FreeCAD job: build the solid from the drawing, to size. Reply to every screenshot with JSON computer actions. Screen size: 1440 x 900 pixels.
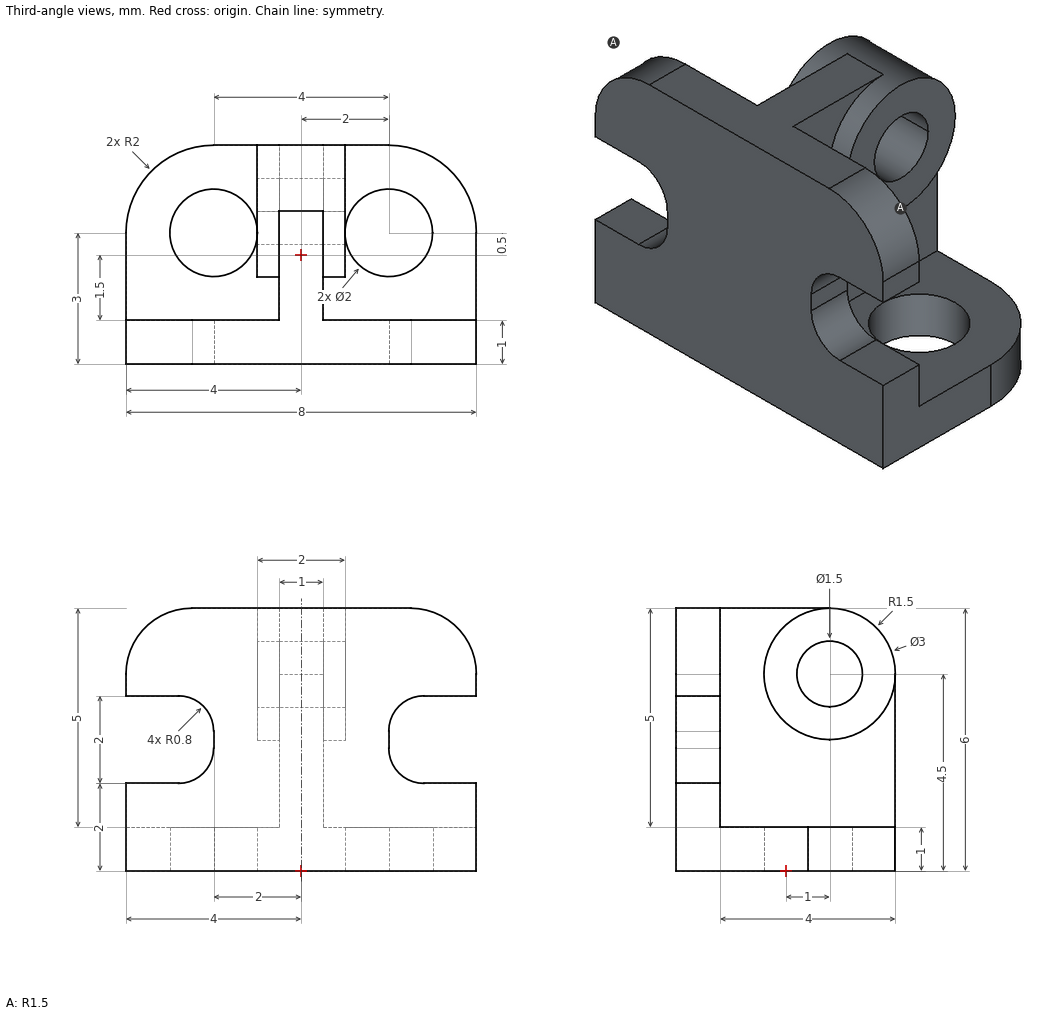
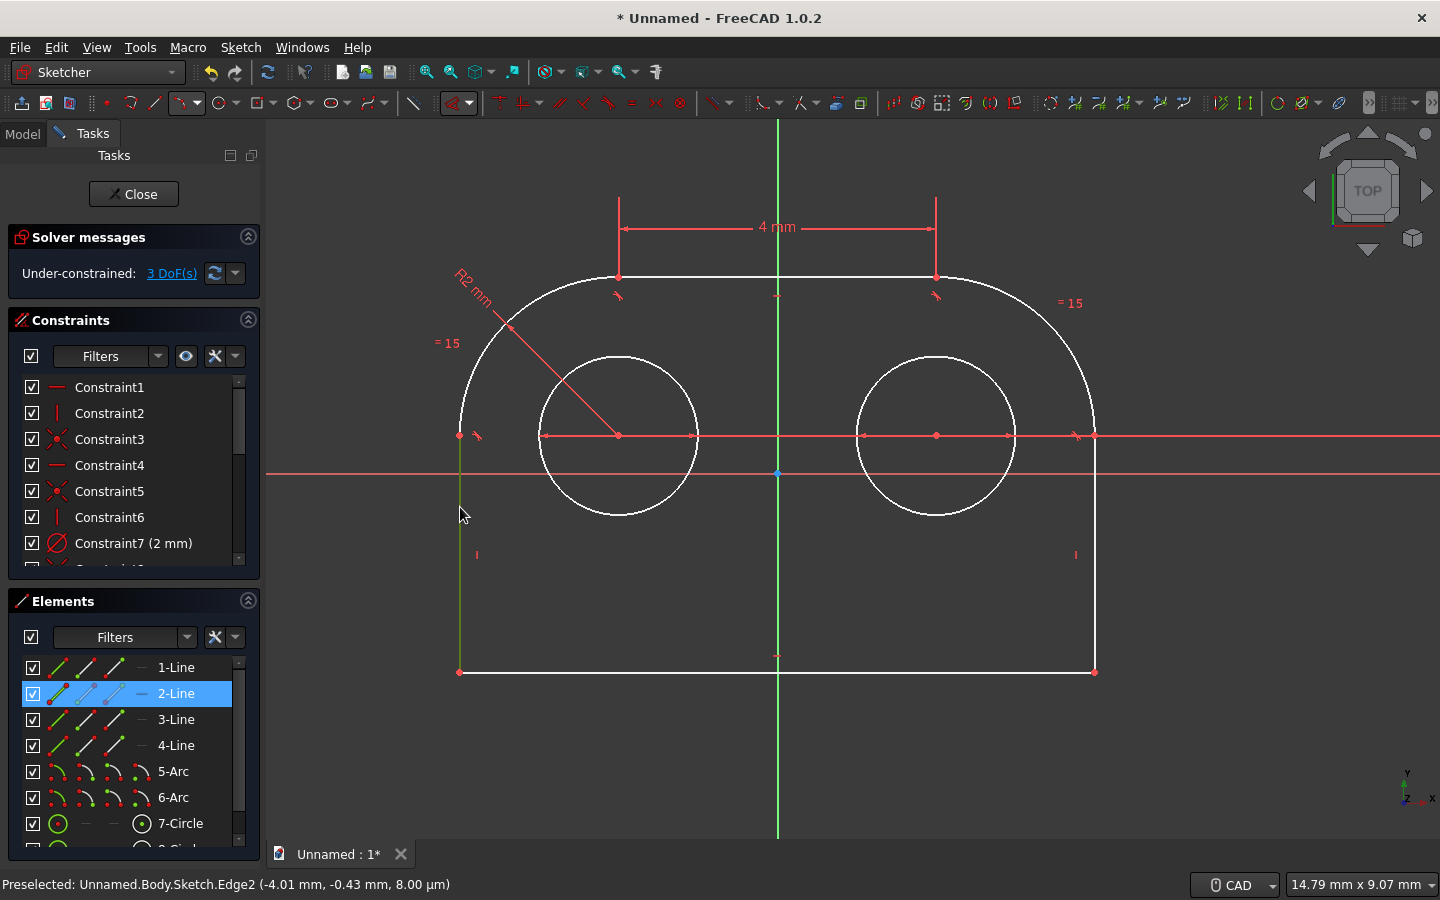
{"action": "key", "text": "i"}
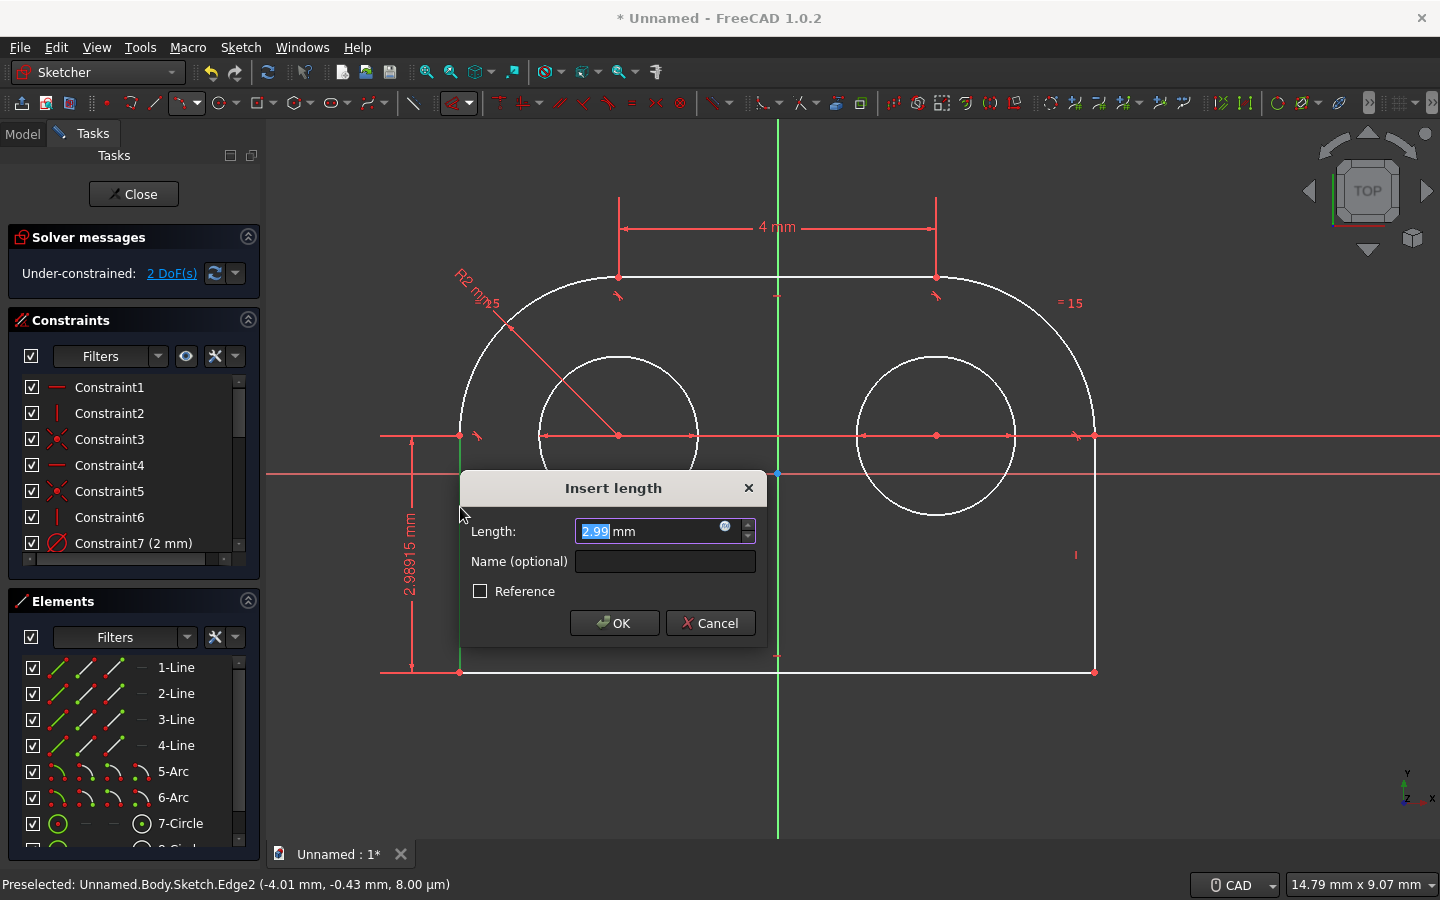
{"action": "type", "text": "3"}
{"action": "key", "text": "Return"}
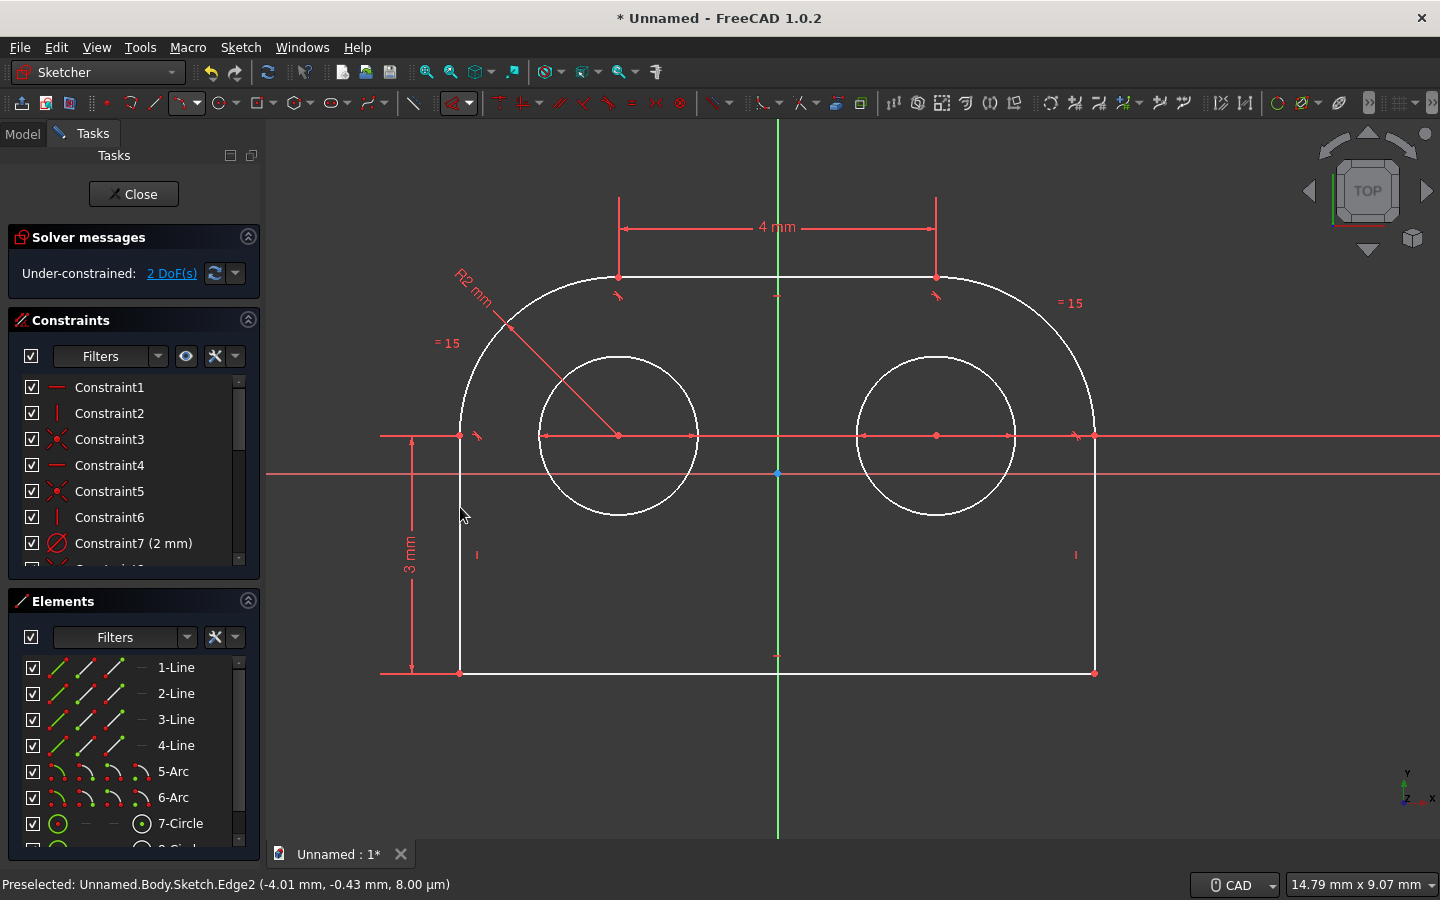
{"action": "left_click", "coordinate": [936, 436]}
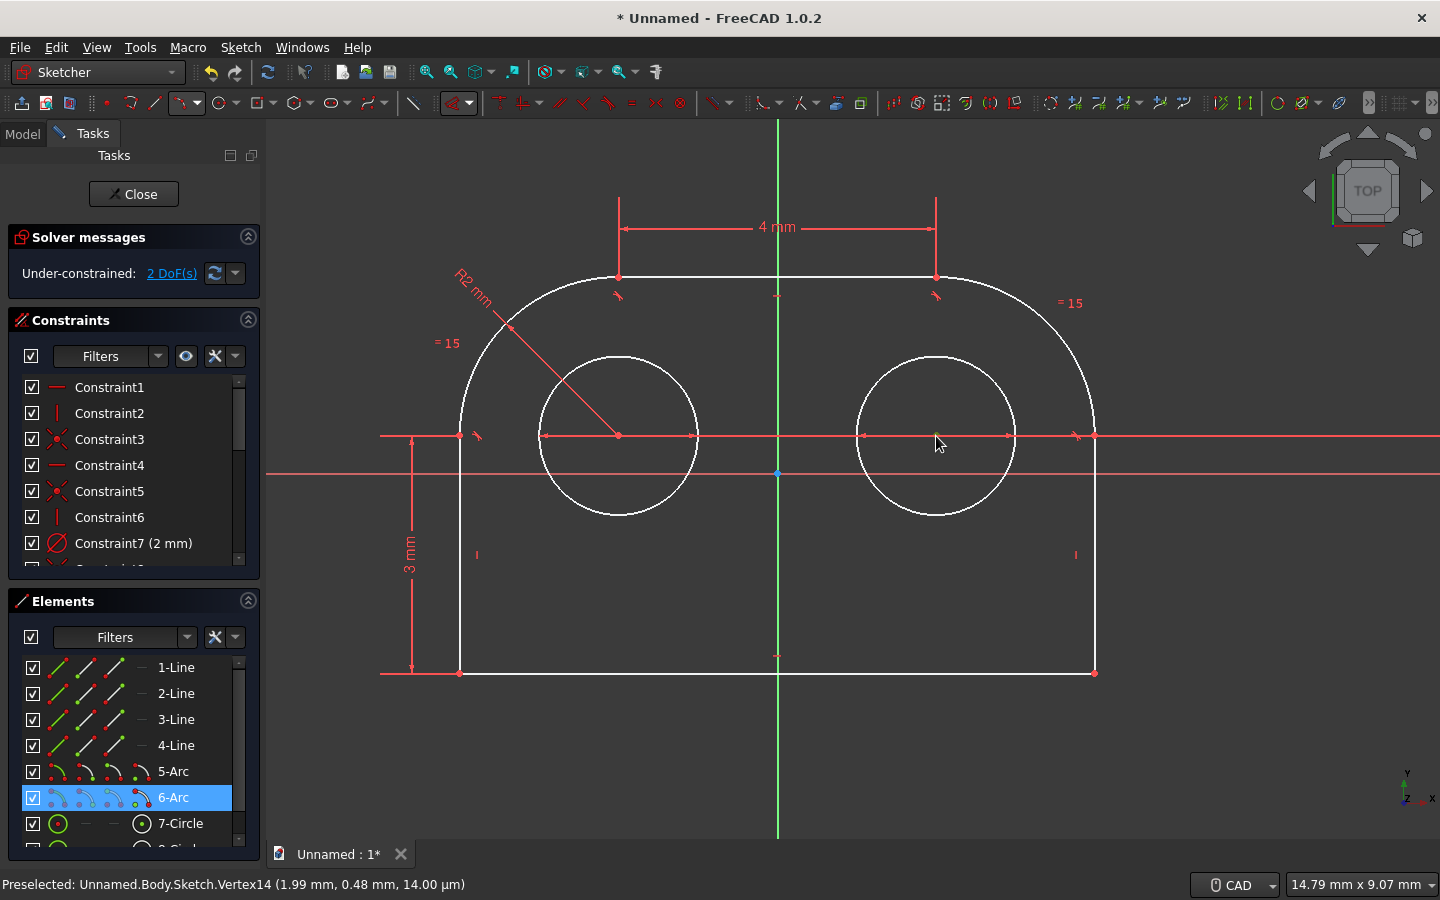
{"action": "key", "text": "l"}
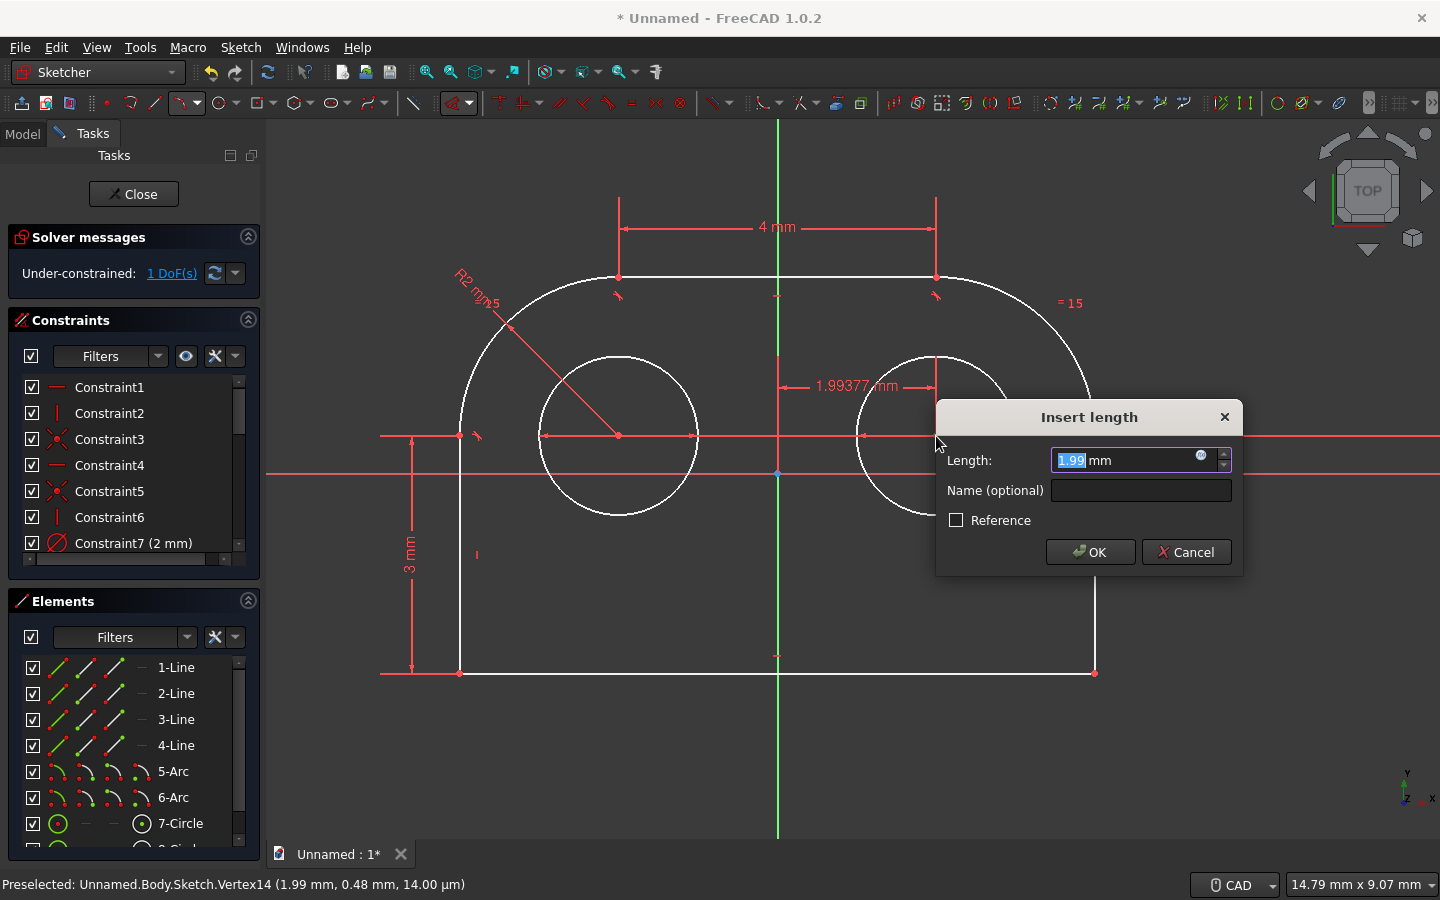
{"action": "type", "text": "2"}
{"action": "key", "text": "Return"}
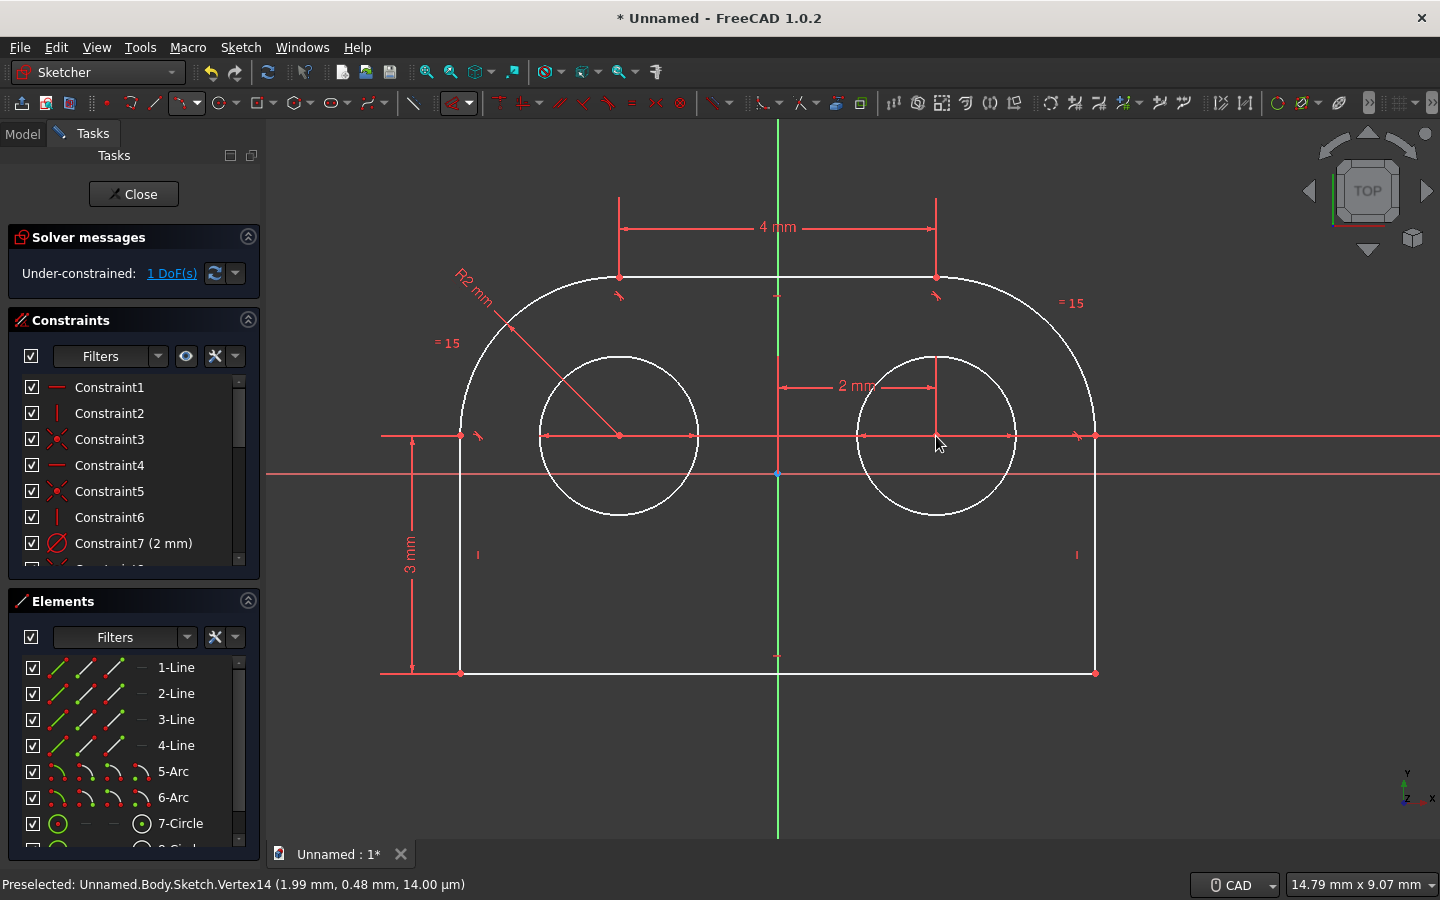
{"action": "left_click", "coordinate": [936, 436]}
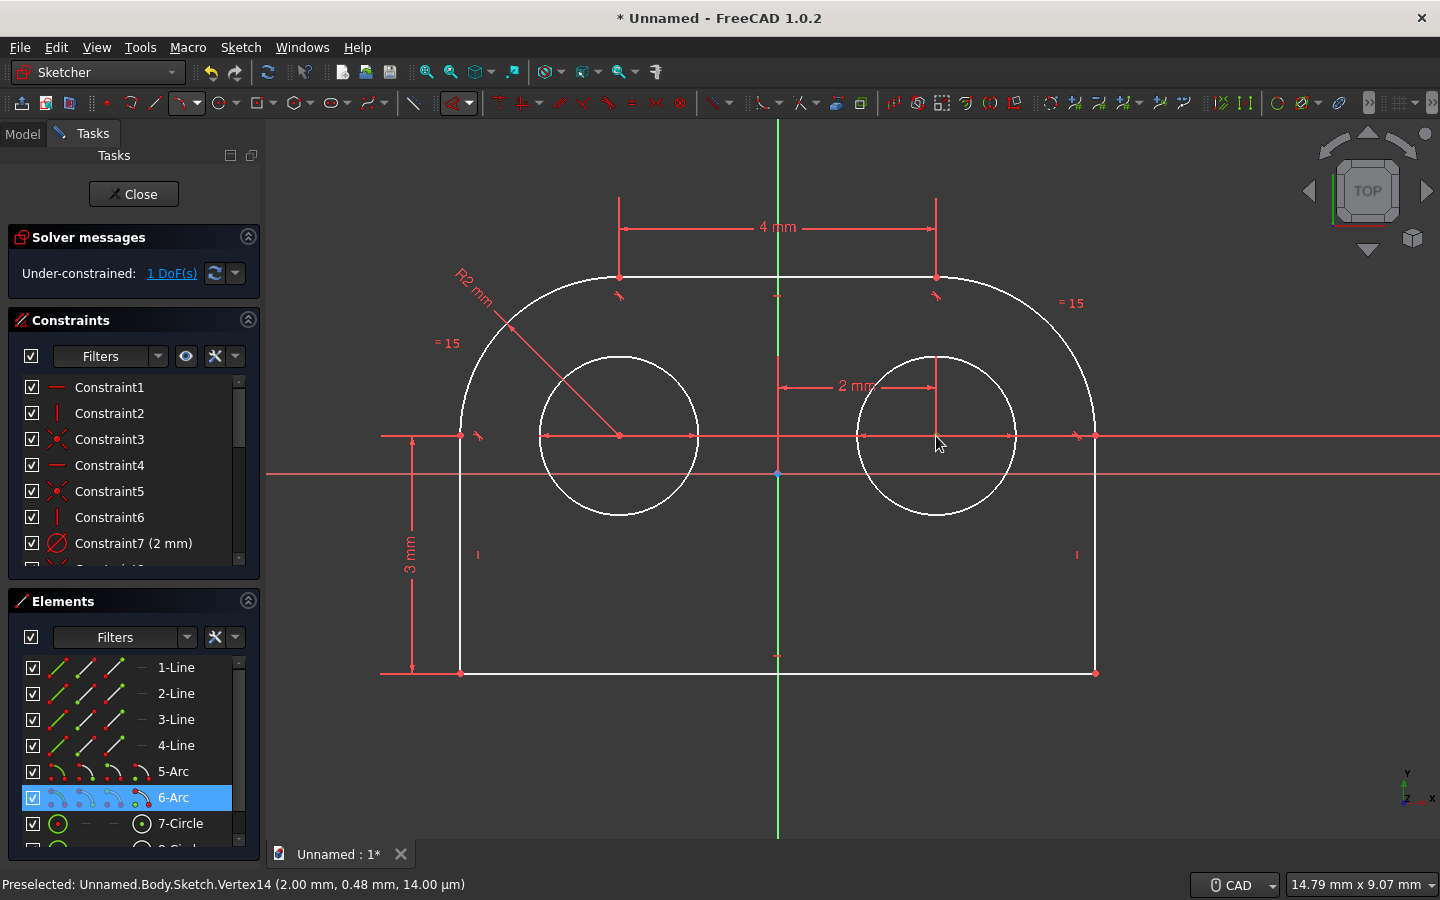
{"action": "left_click", "coordinate": [472, 104]}